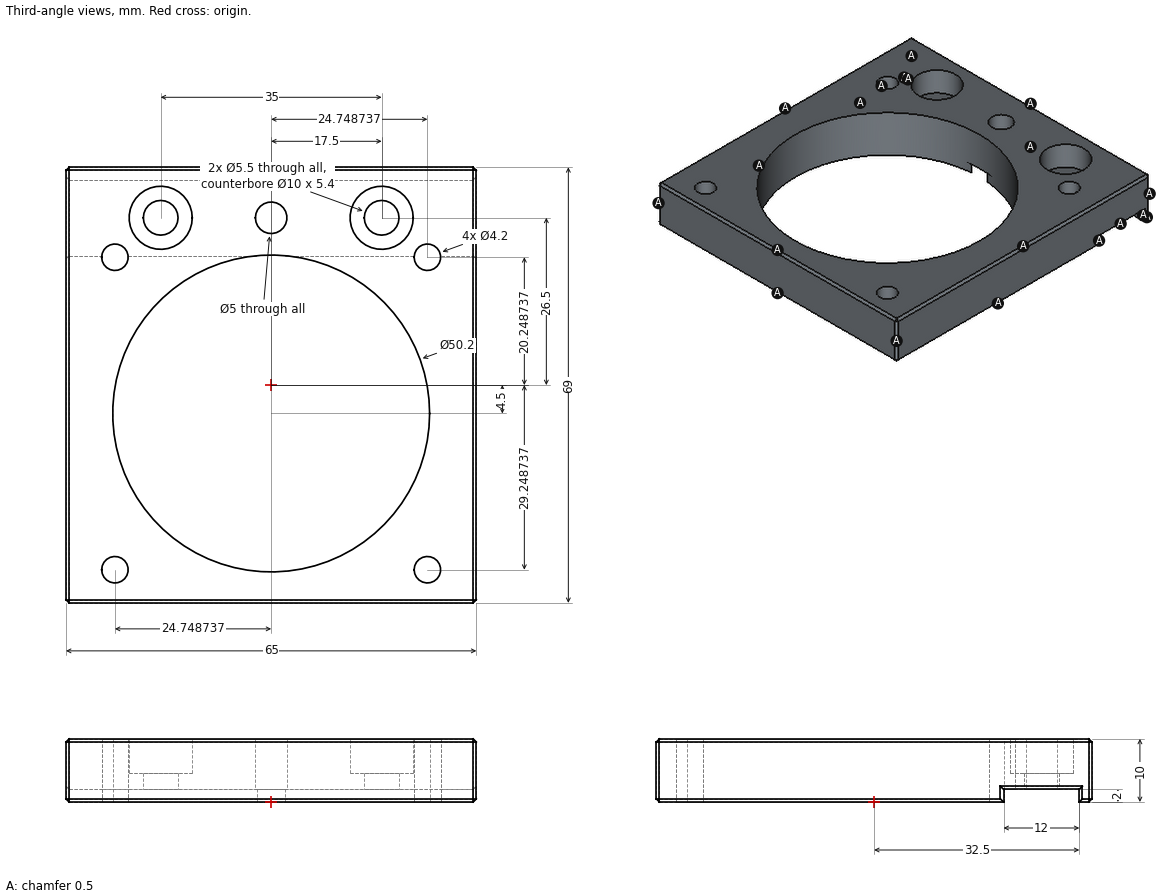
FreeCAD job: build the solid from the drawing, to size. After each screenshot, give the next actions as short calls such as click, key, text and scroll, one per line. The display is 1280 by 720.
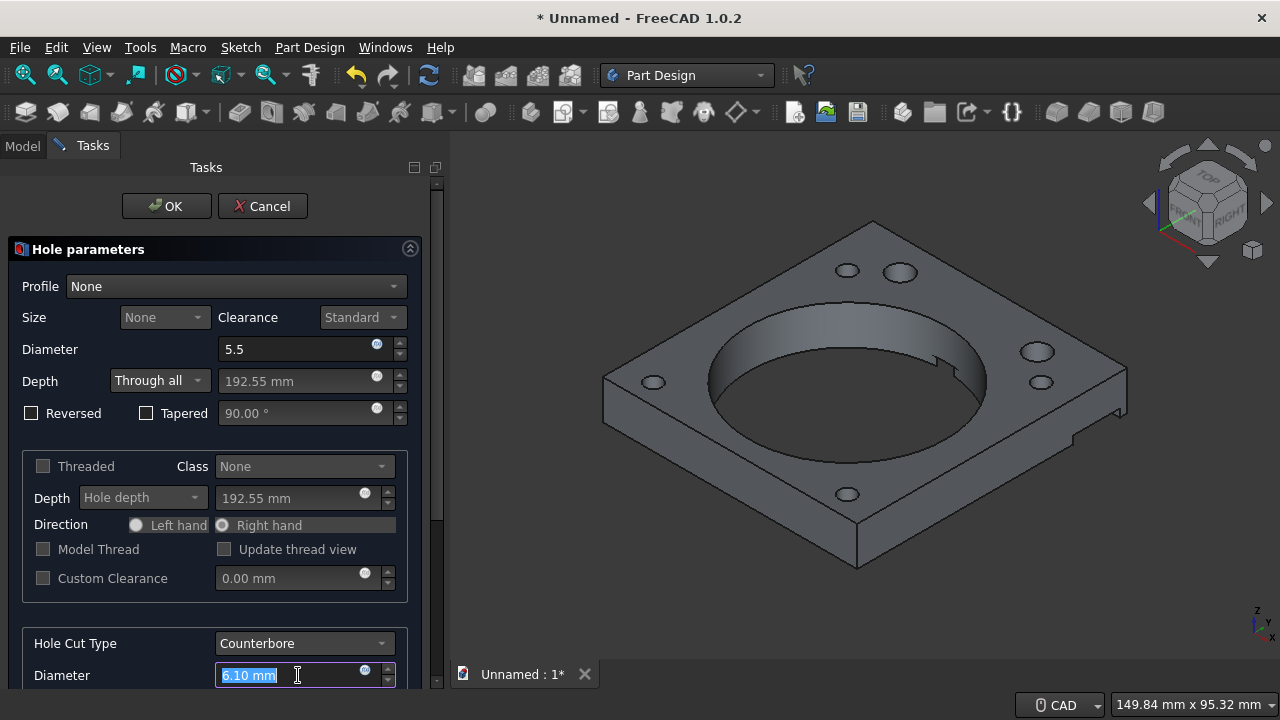
text(10)
key(Tab)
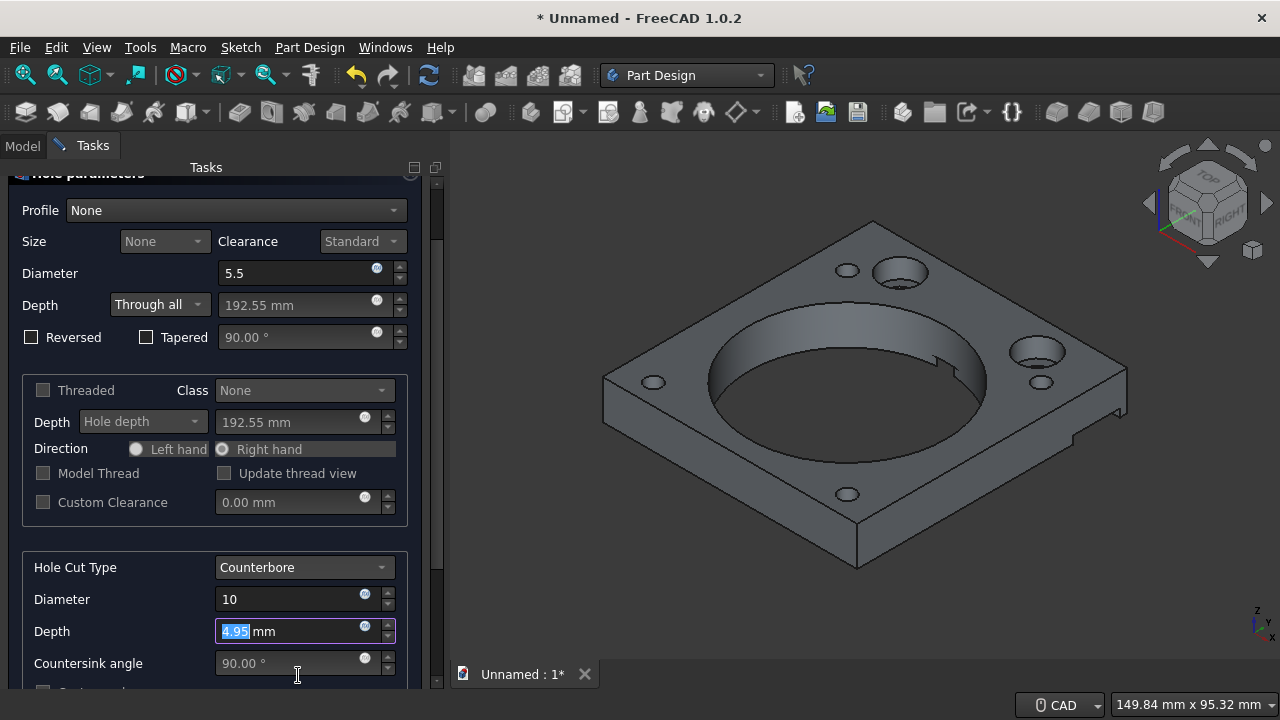
text(5.4)
key(Tab)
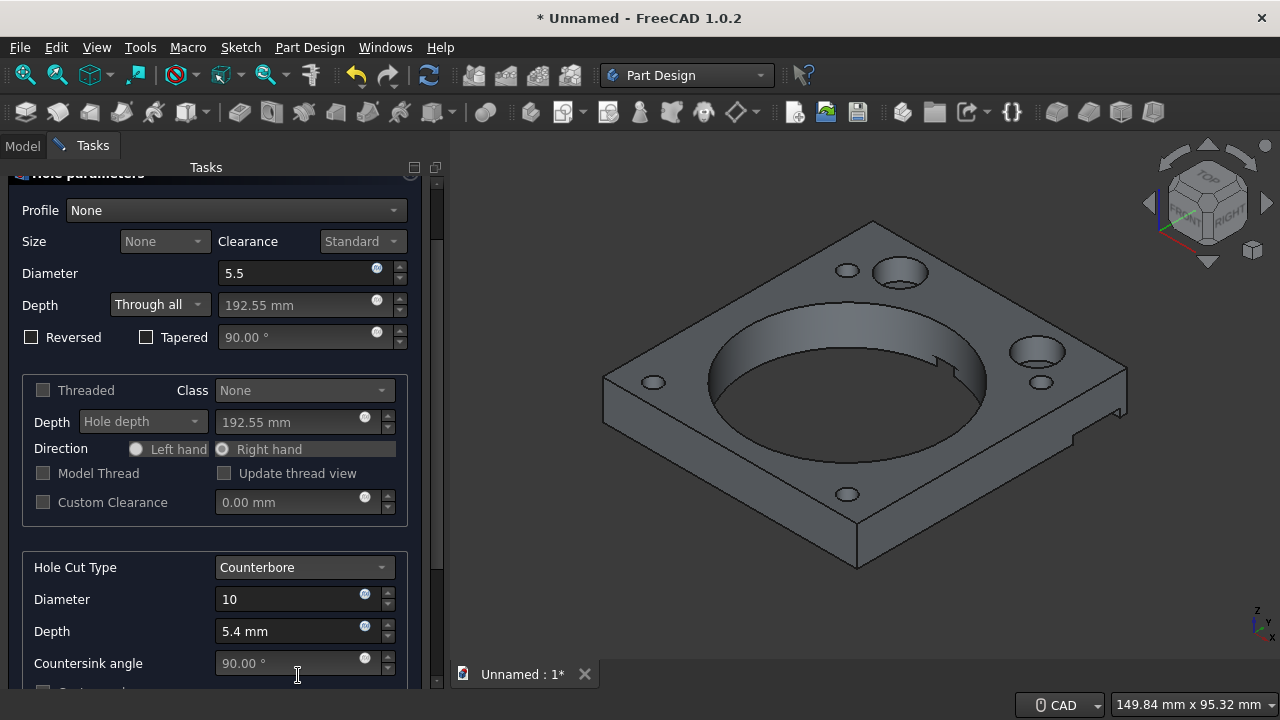
scroll(437, 432, up, 3)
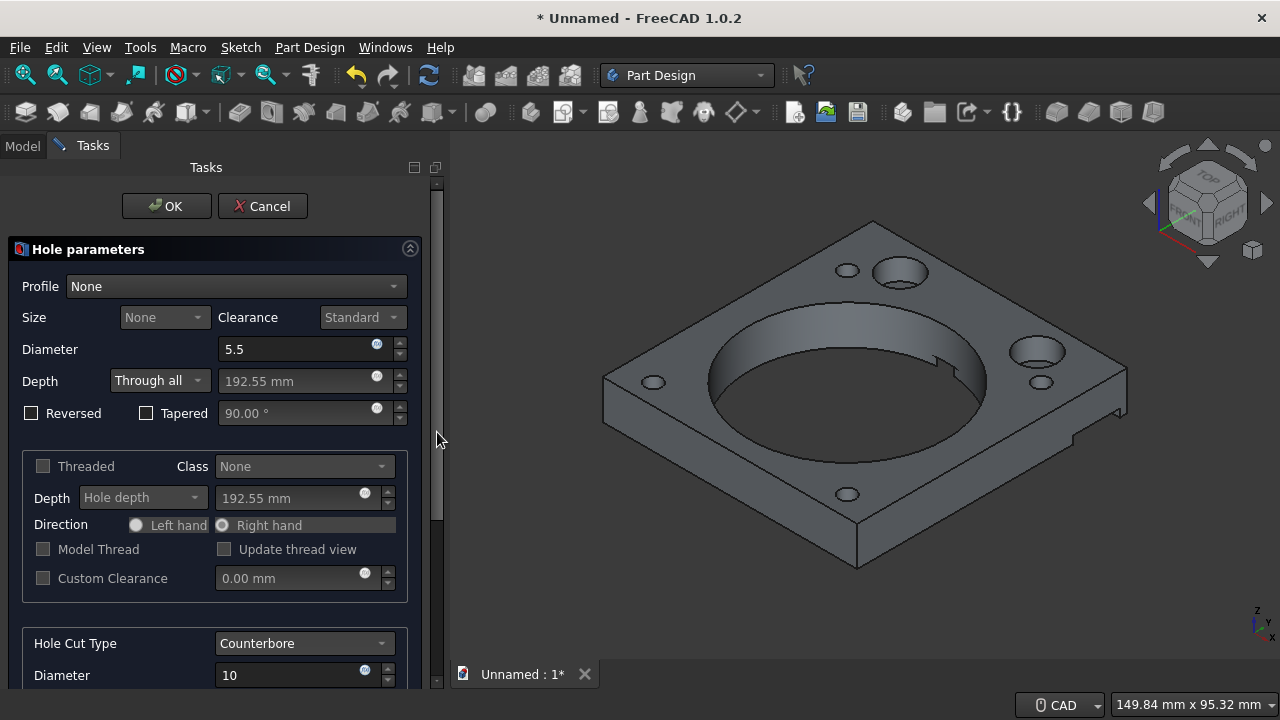
click(167, 206)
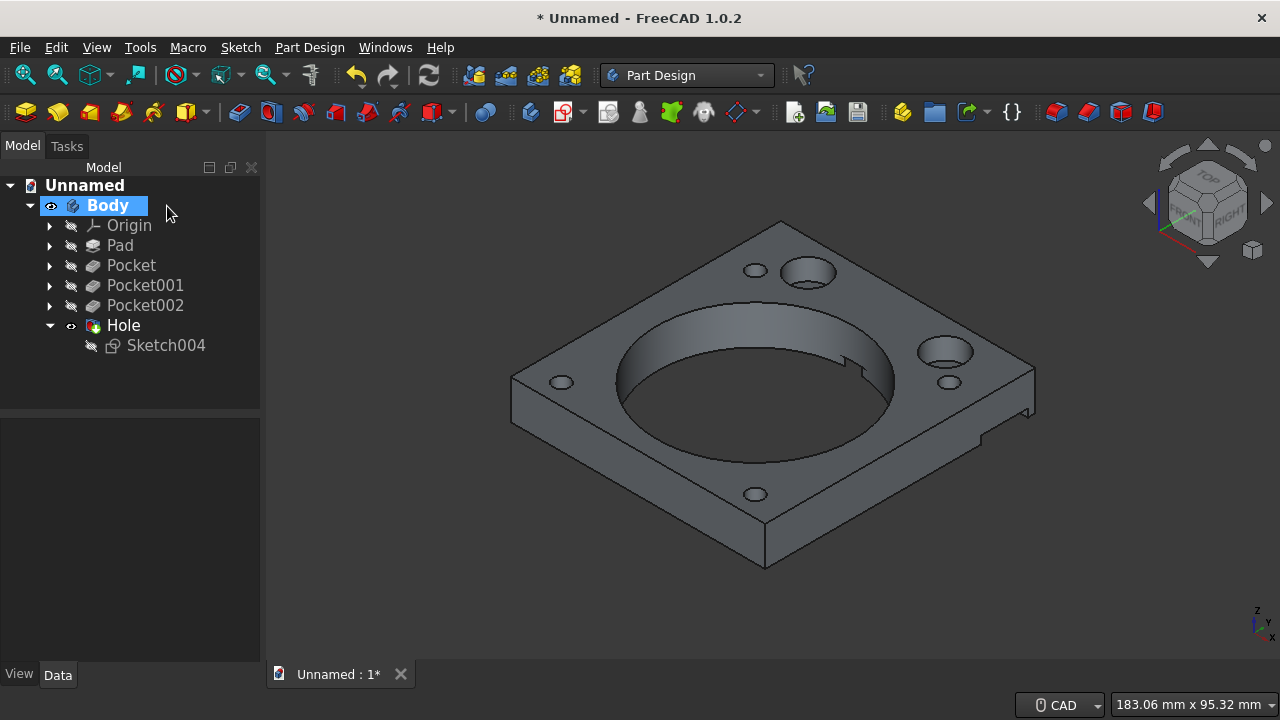
click(889, 305)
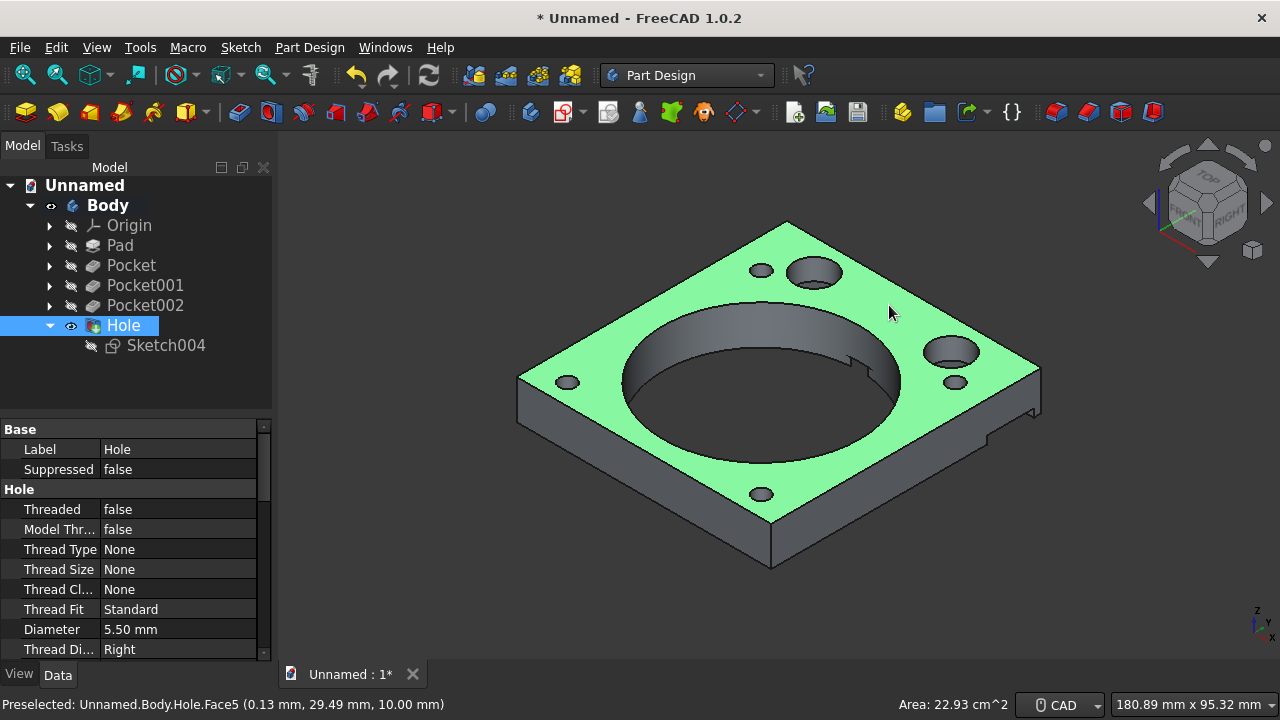
click(564, 112)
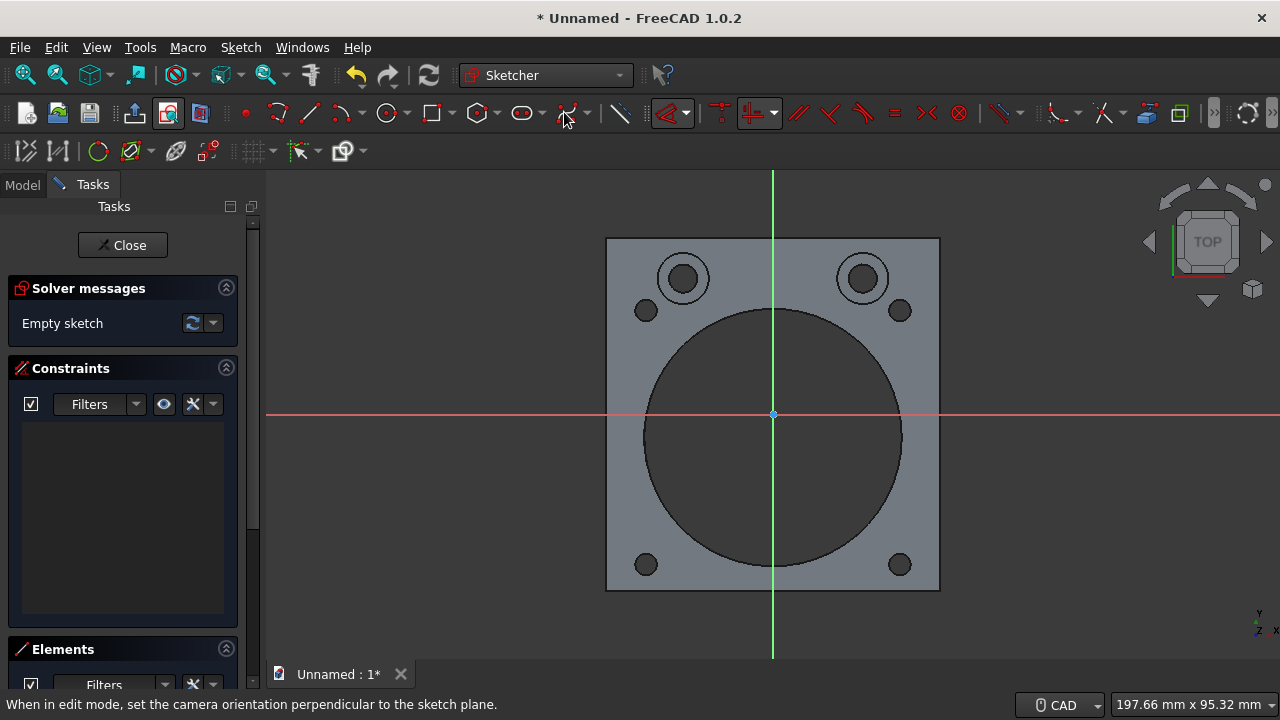
scroll(780, 265, up, 12)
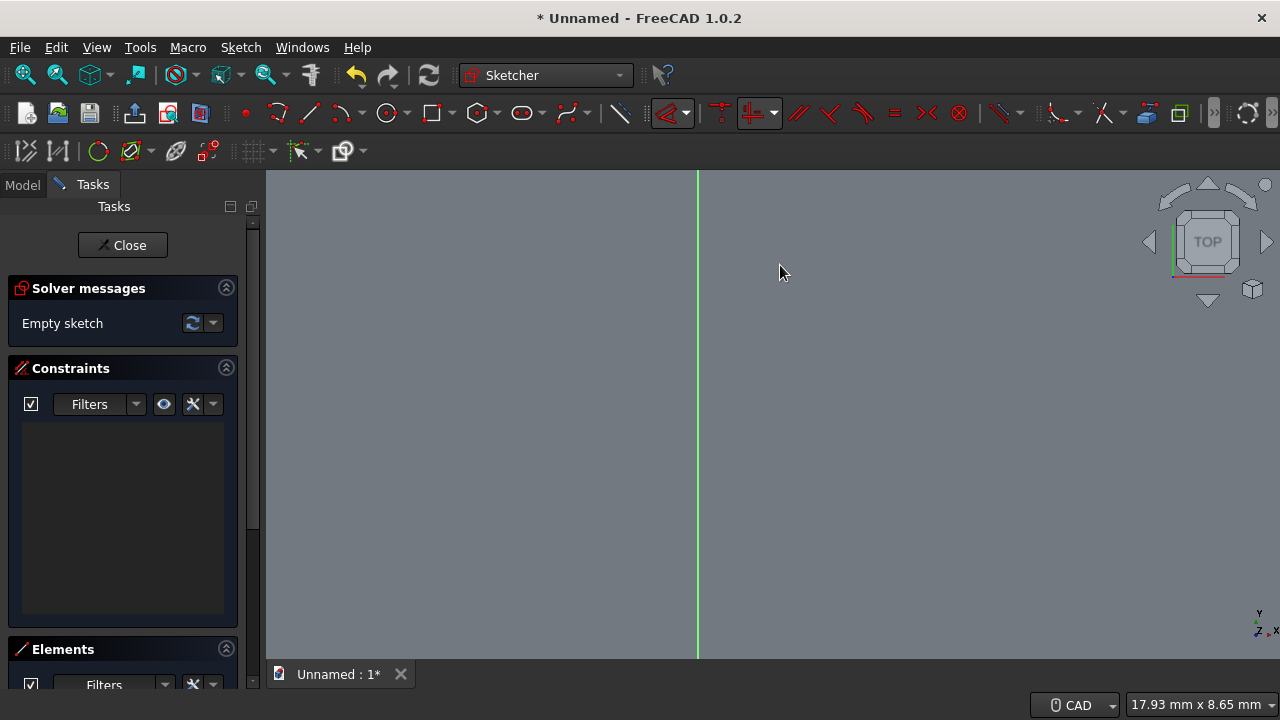
click(388, 114)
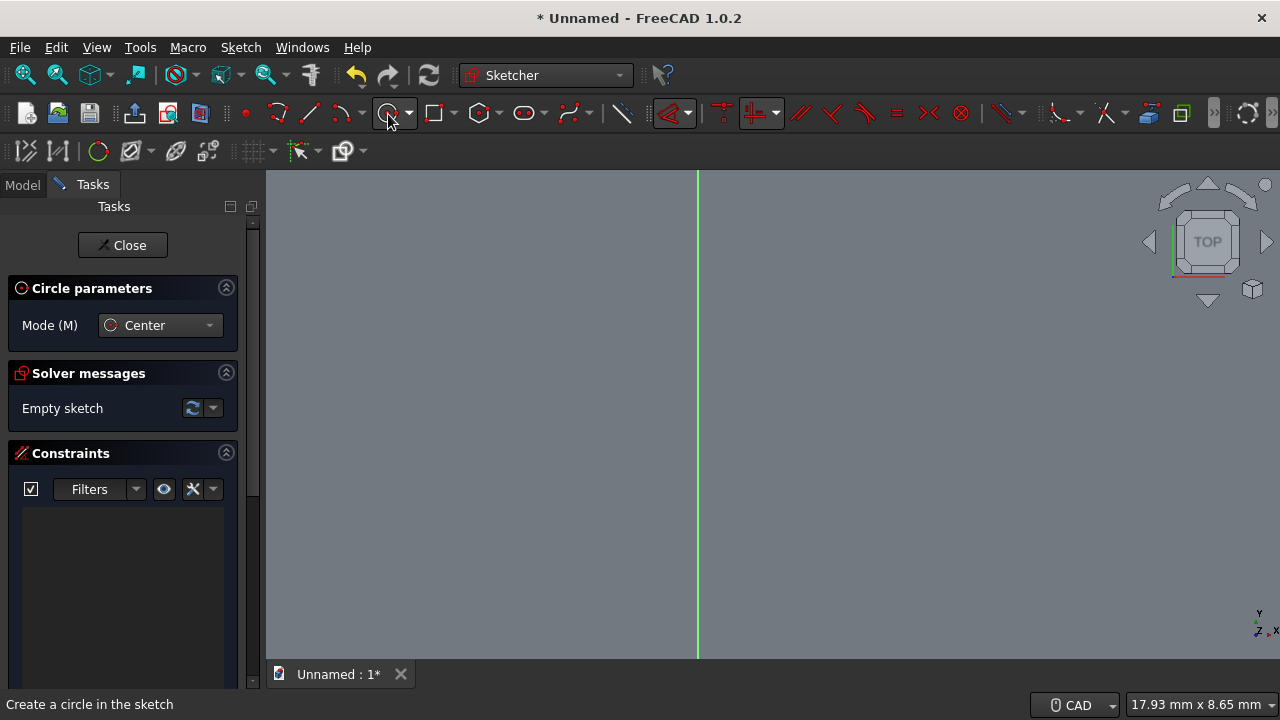
click(698, 412)
click(798, 312)
key(Escape)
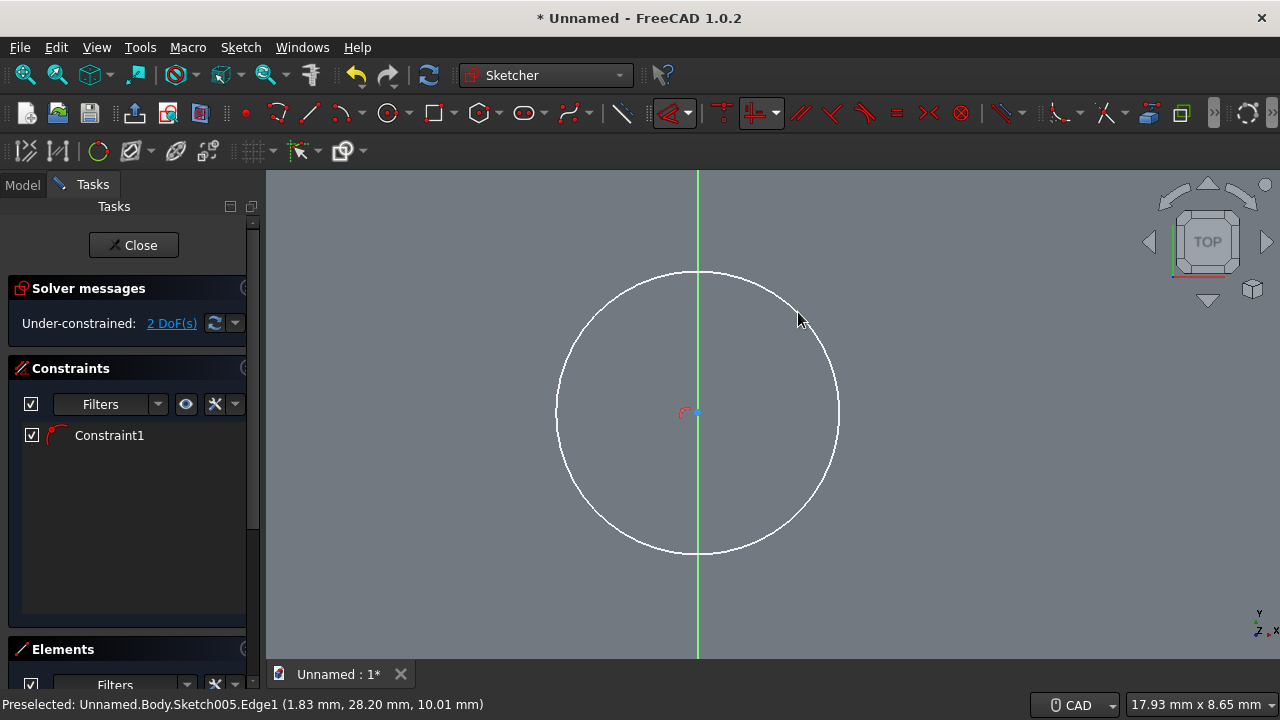
click(798, 313)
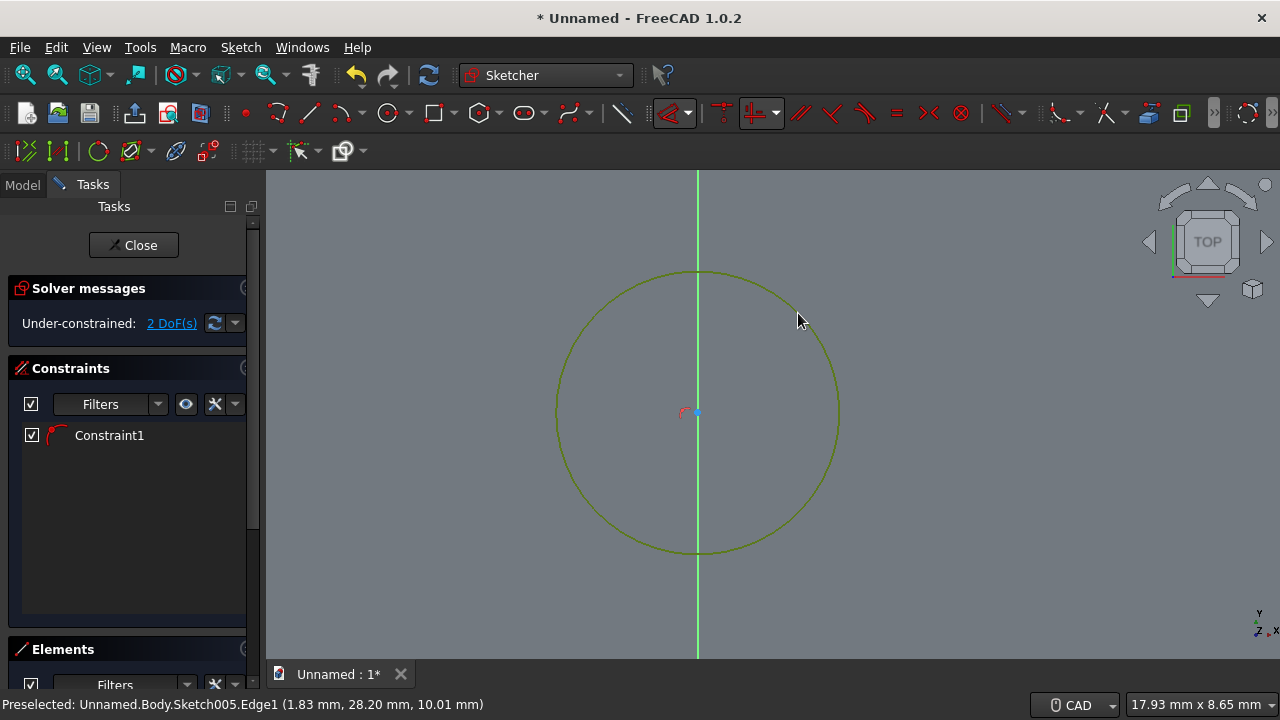
key(k)
key(o)